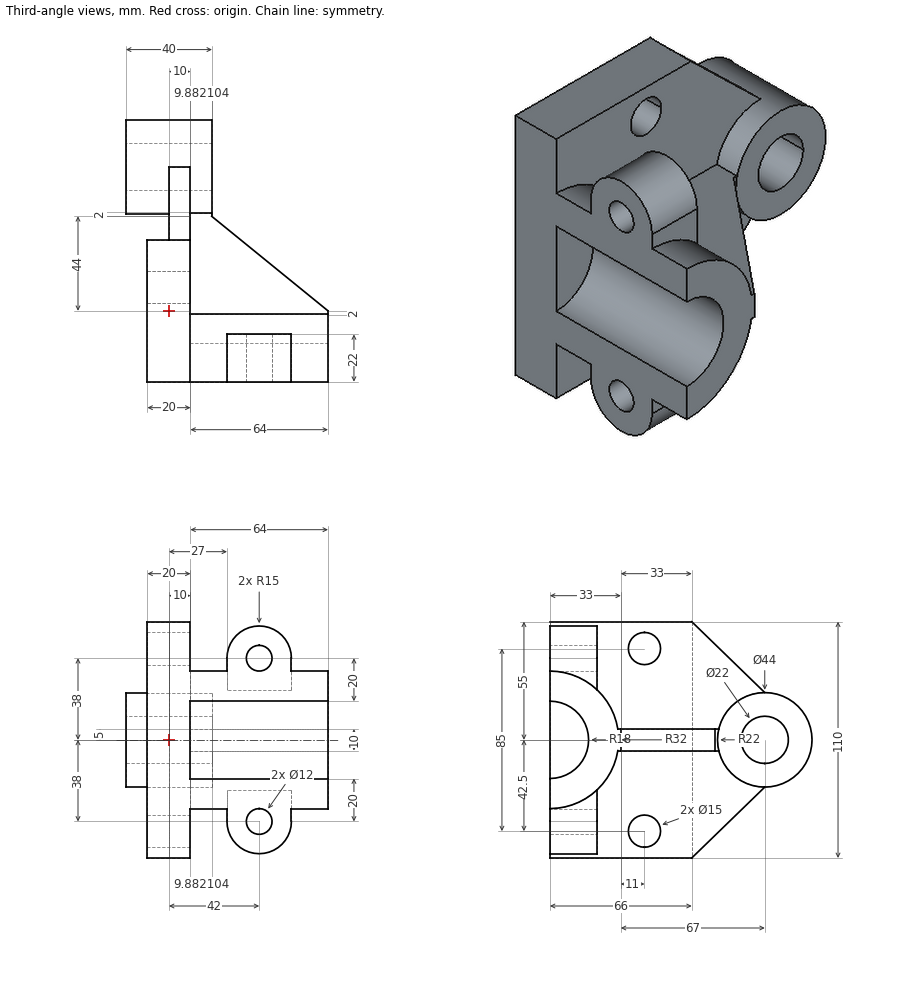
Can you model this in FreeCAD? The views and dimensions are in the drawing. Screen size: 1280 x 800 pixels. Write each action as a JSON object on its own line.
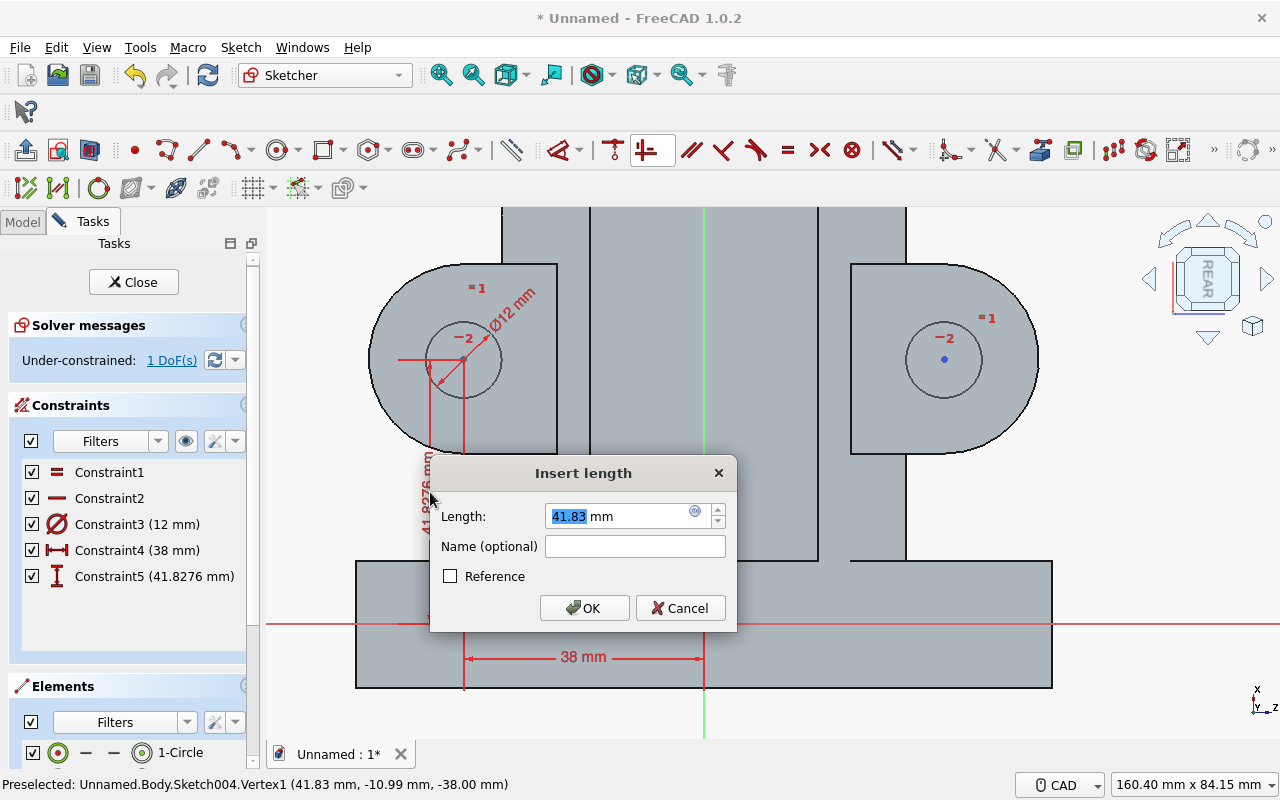
{"action": "type", "text": "42"}
{"action": "key", "text": "Return"}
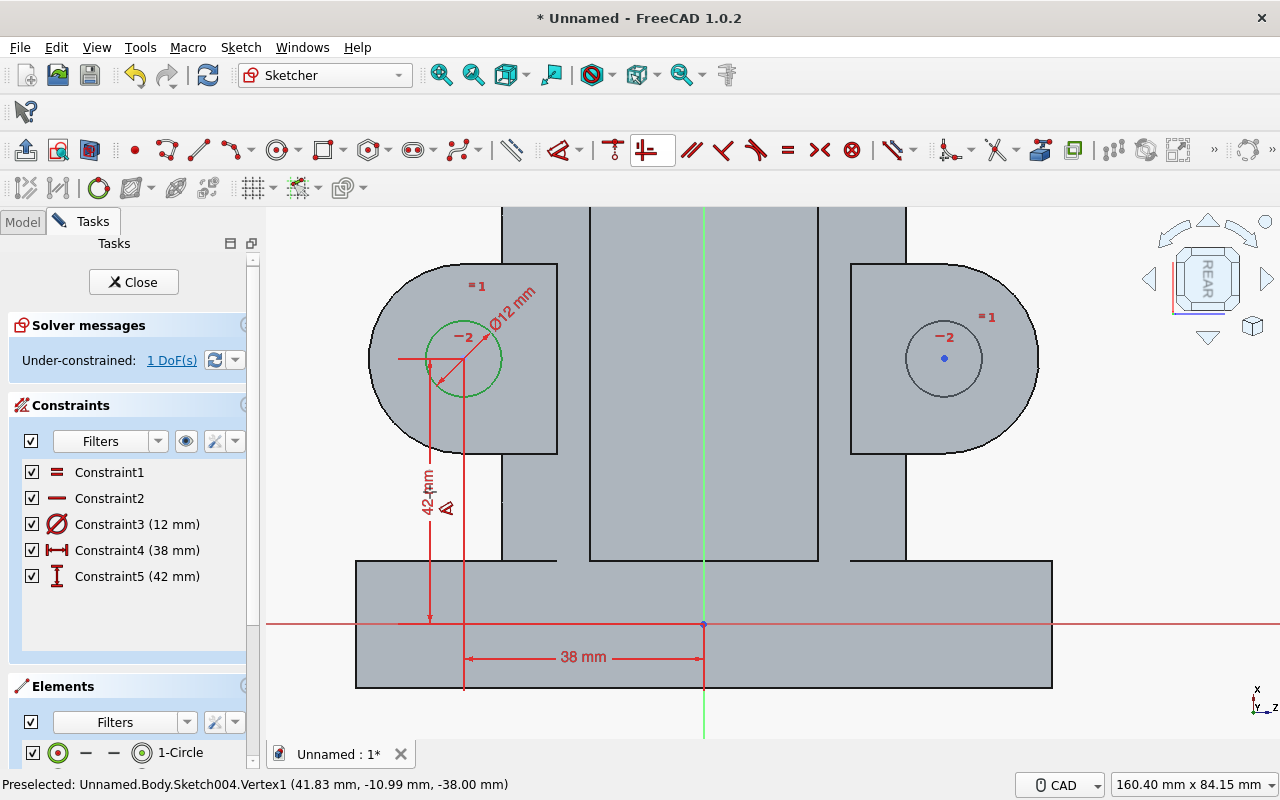
{"action": "left_click", "coordinate": [944, 359]}
{"action": "left_click", "coordinate": [824, 658]}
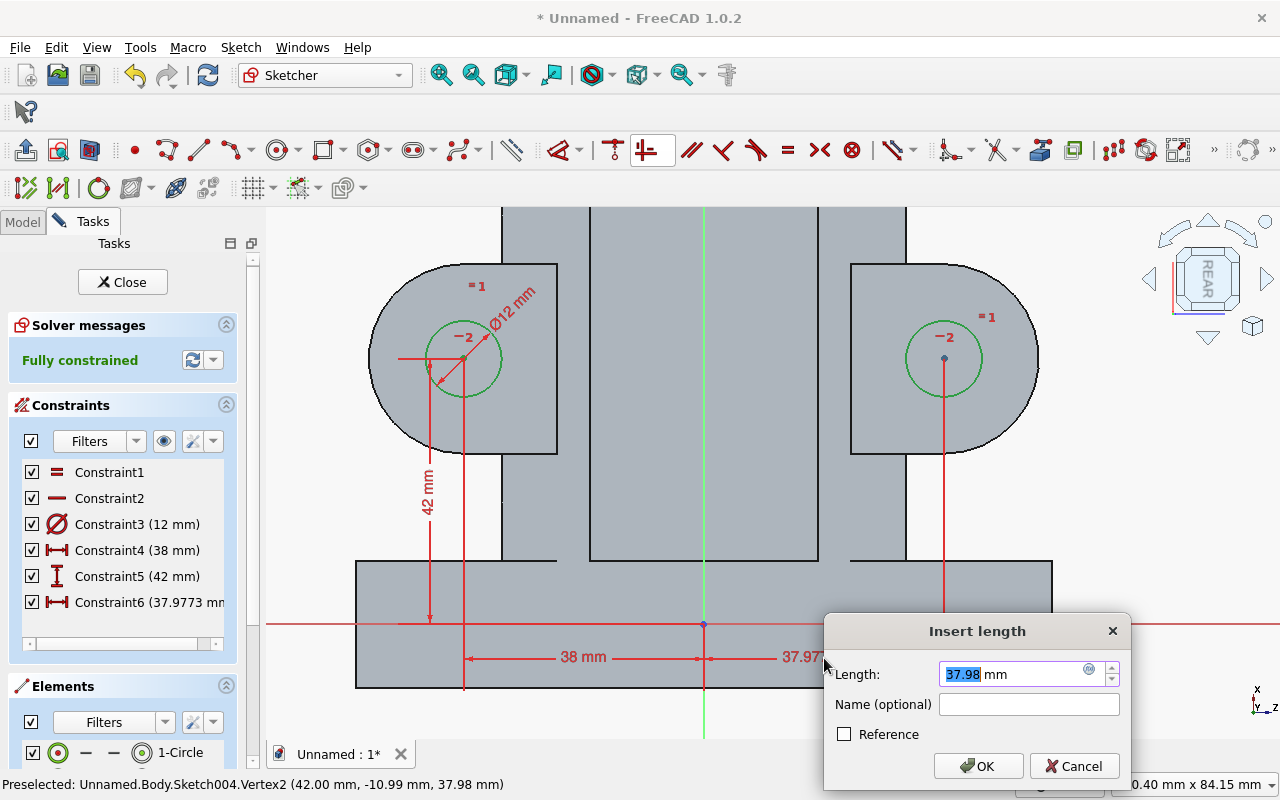
{"action": "type", "text": "38"}
{"action": "key", "text": "Return"}
{"action": "key", "text": "Escape"}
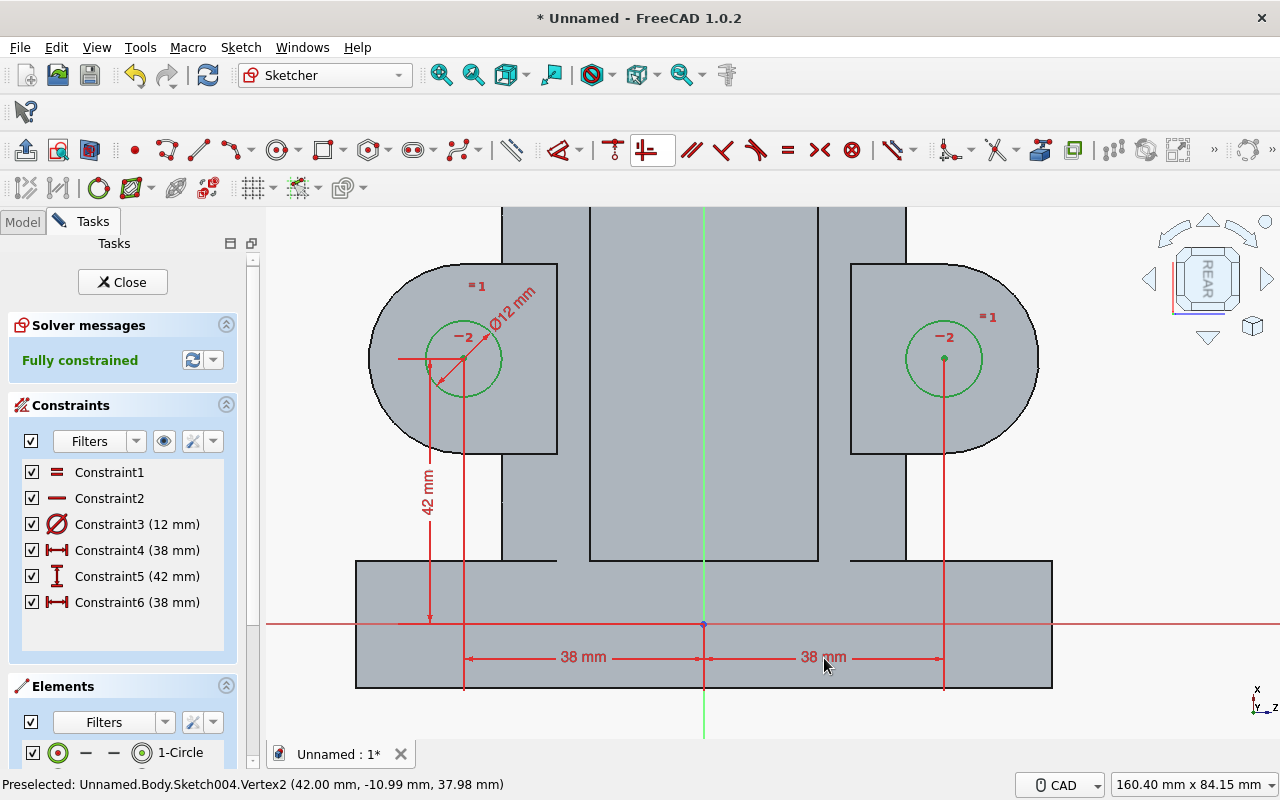
{"action": "left_click", "coordinate": [123, 282]}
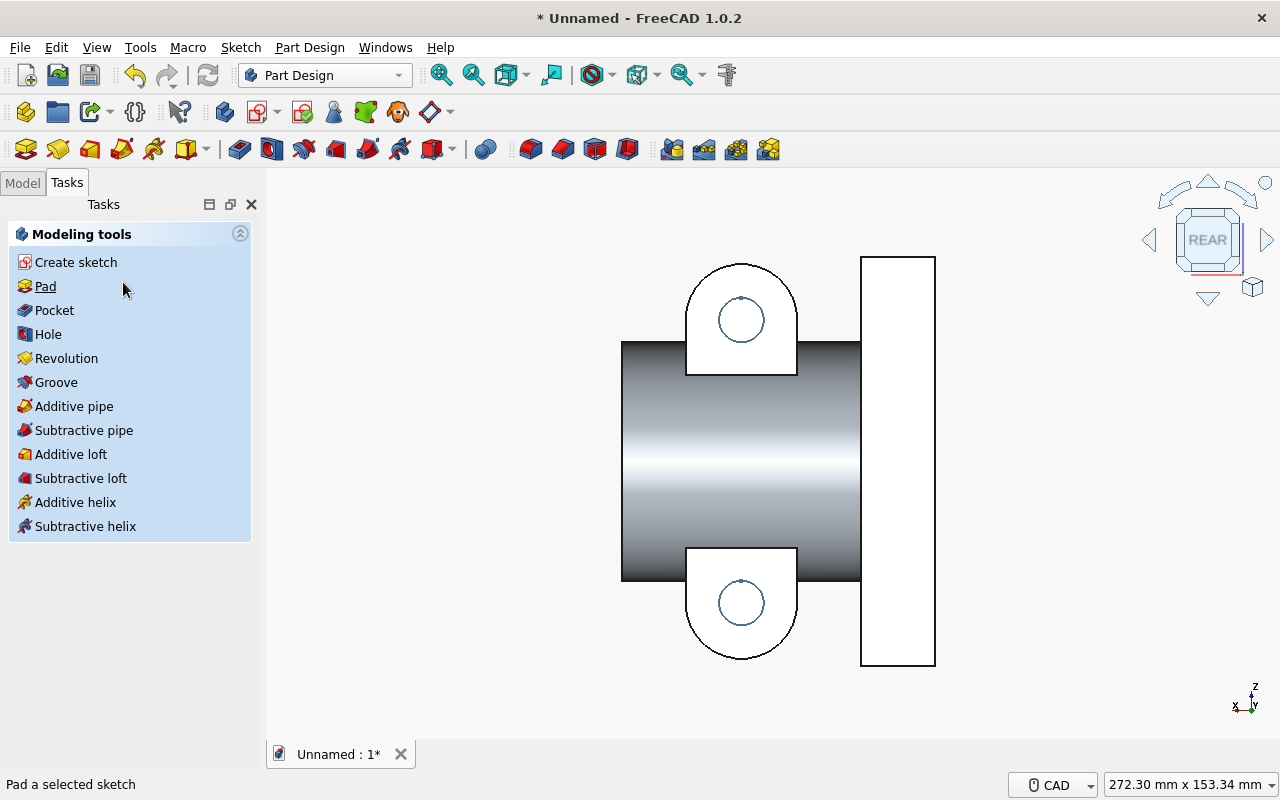
{"action": "left_click", "coordinate": [240, 150]}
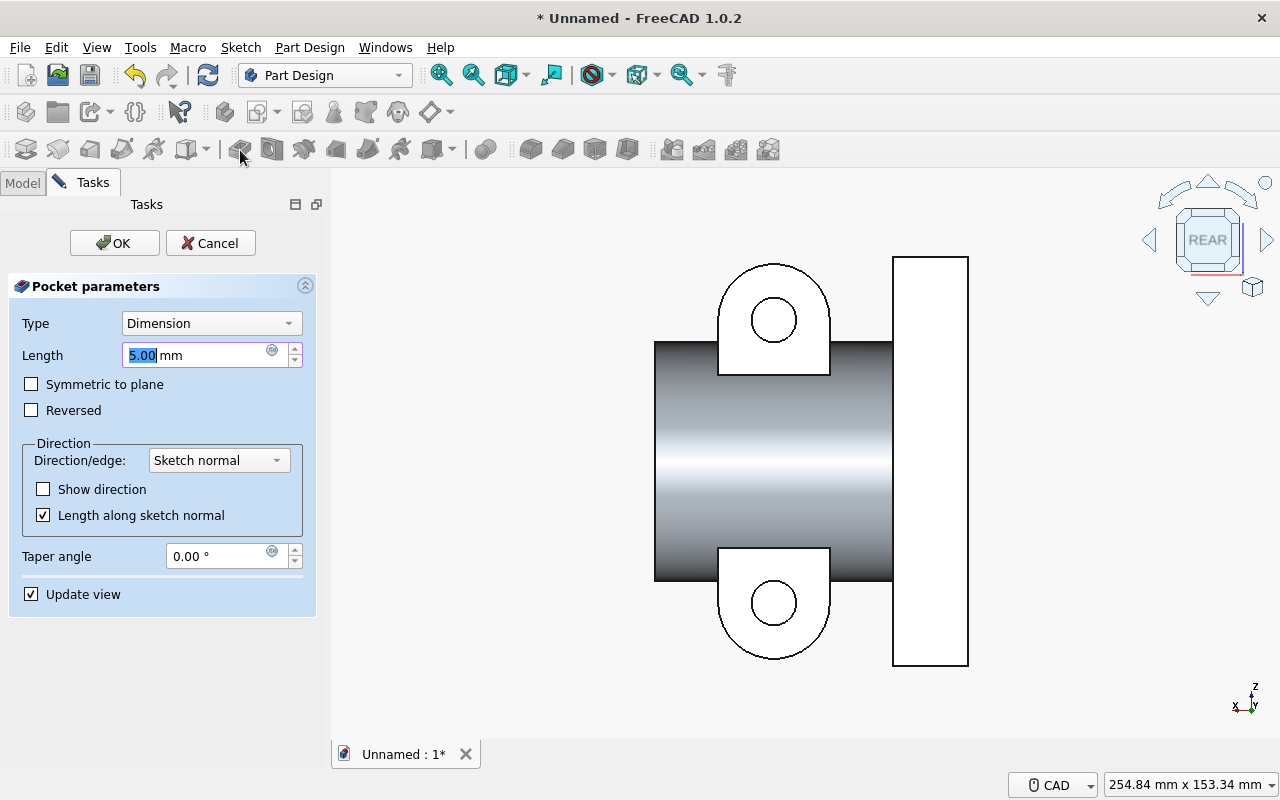
{"action": "type", "text": "22"}
{"action": "key", "text": "Tab"}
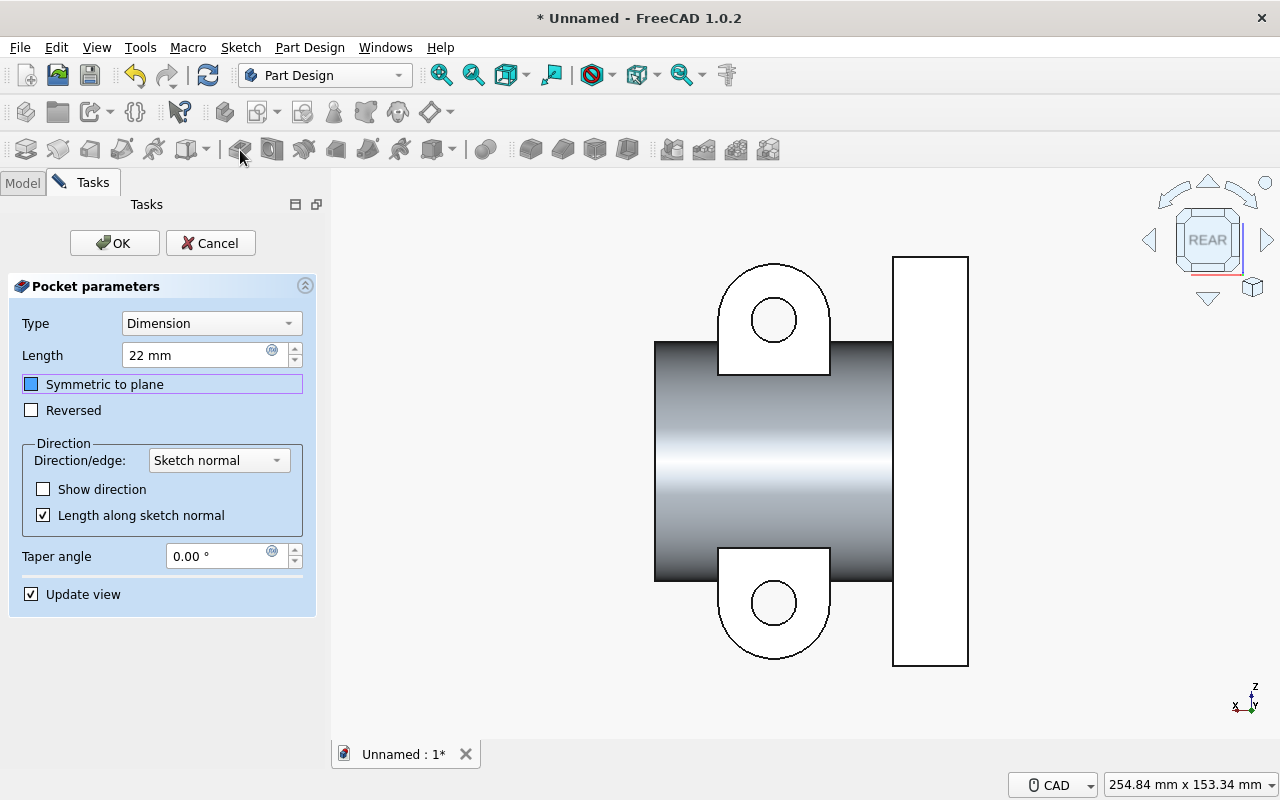
{"action": "left_click", "coordinate": [115, 243]}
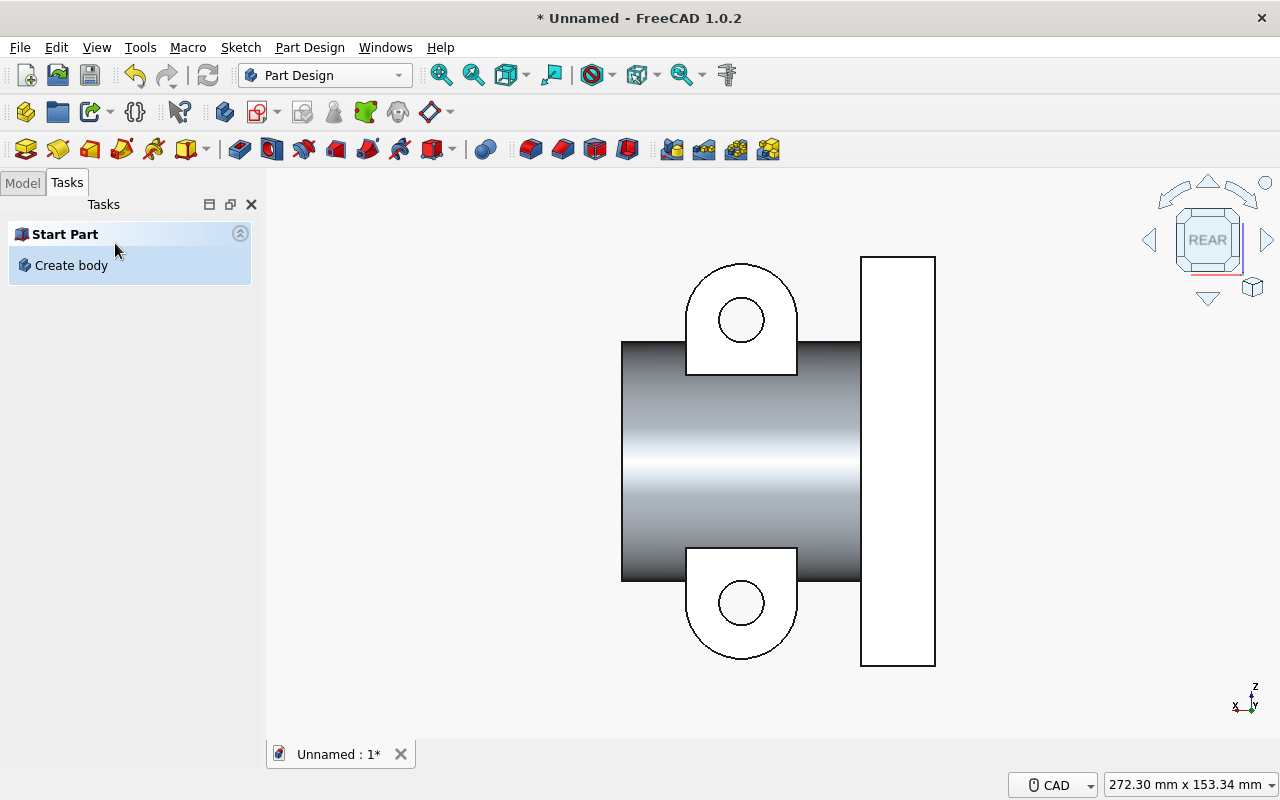
{"action": "left_click", "coordinate": [226, 112]}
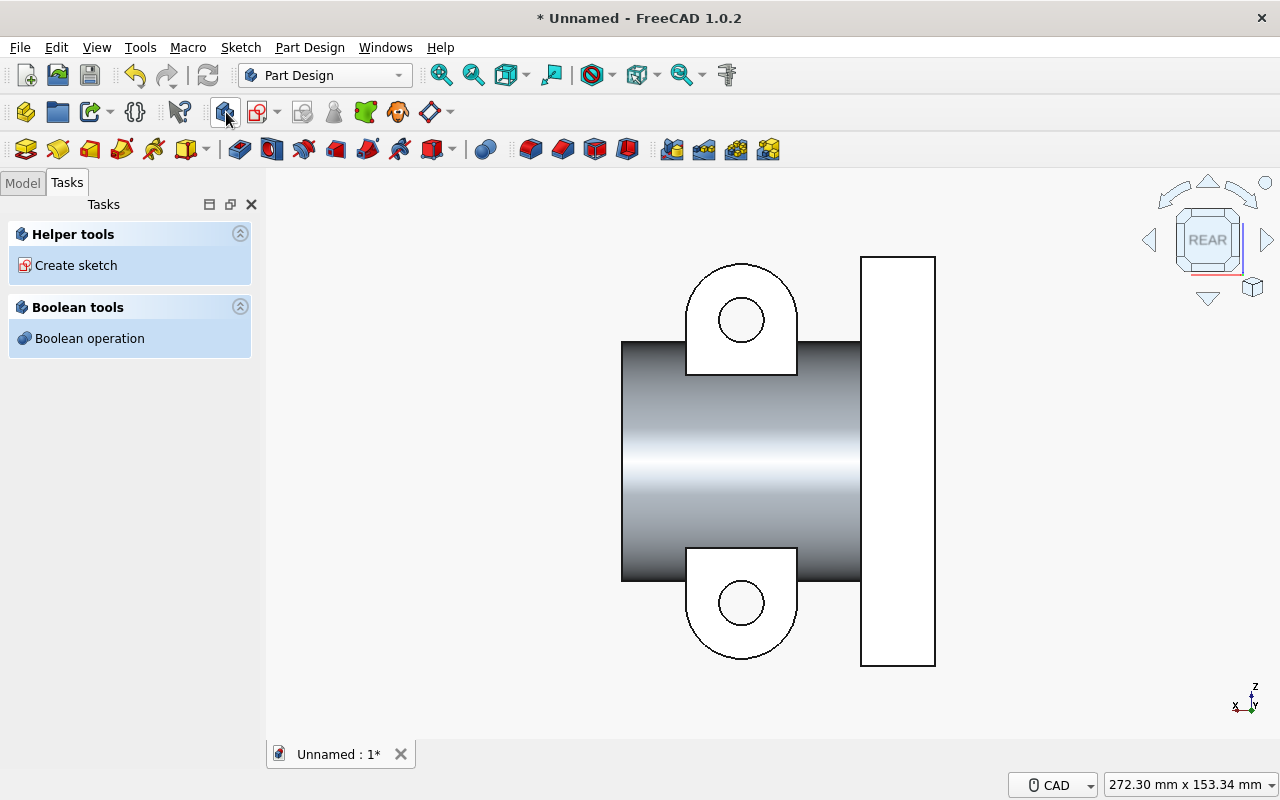
{"action": "left_click", "coordinate": [306, 699]}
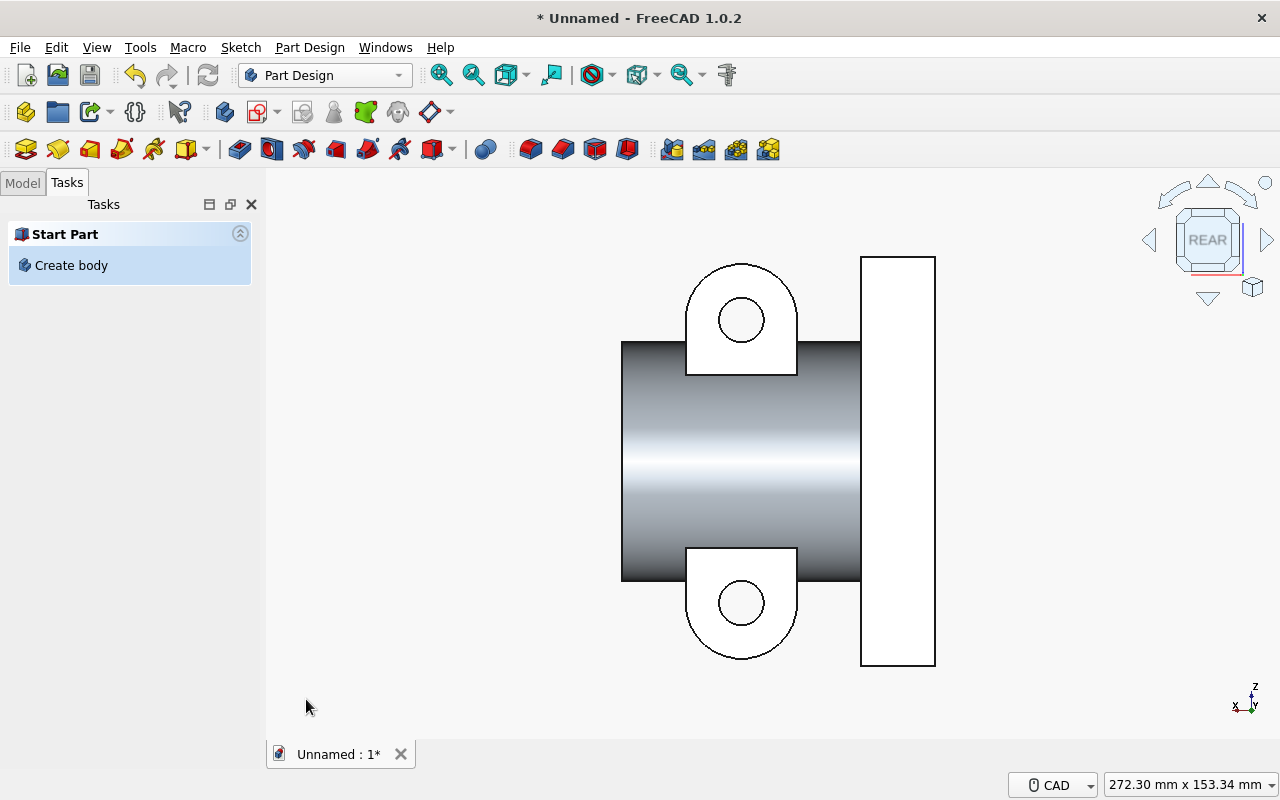
{"action": "left_click", "coordinate": [258, 112]}